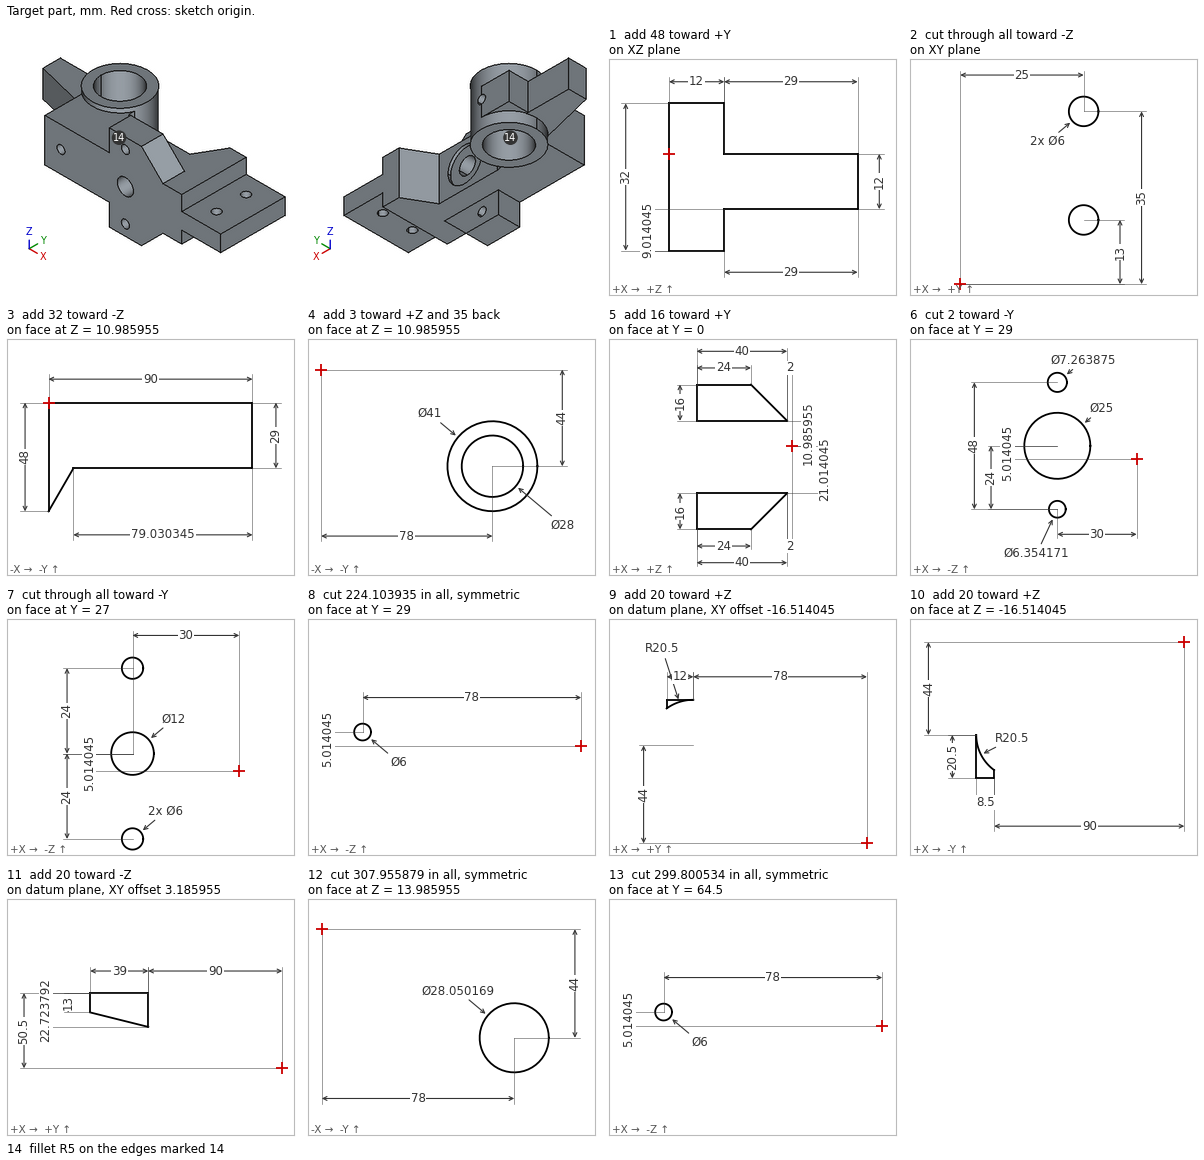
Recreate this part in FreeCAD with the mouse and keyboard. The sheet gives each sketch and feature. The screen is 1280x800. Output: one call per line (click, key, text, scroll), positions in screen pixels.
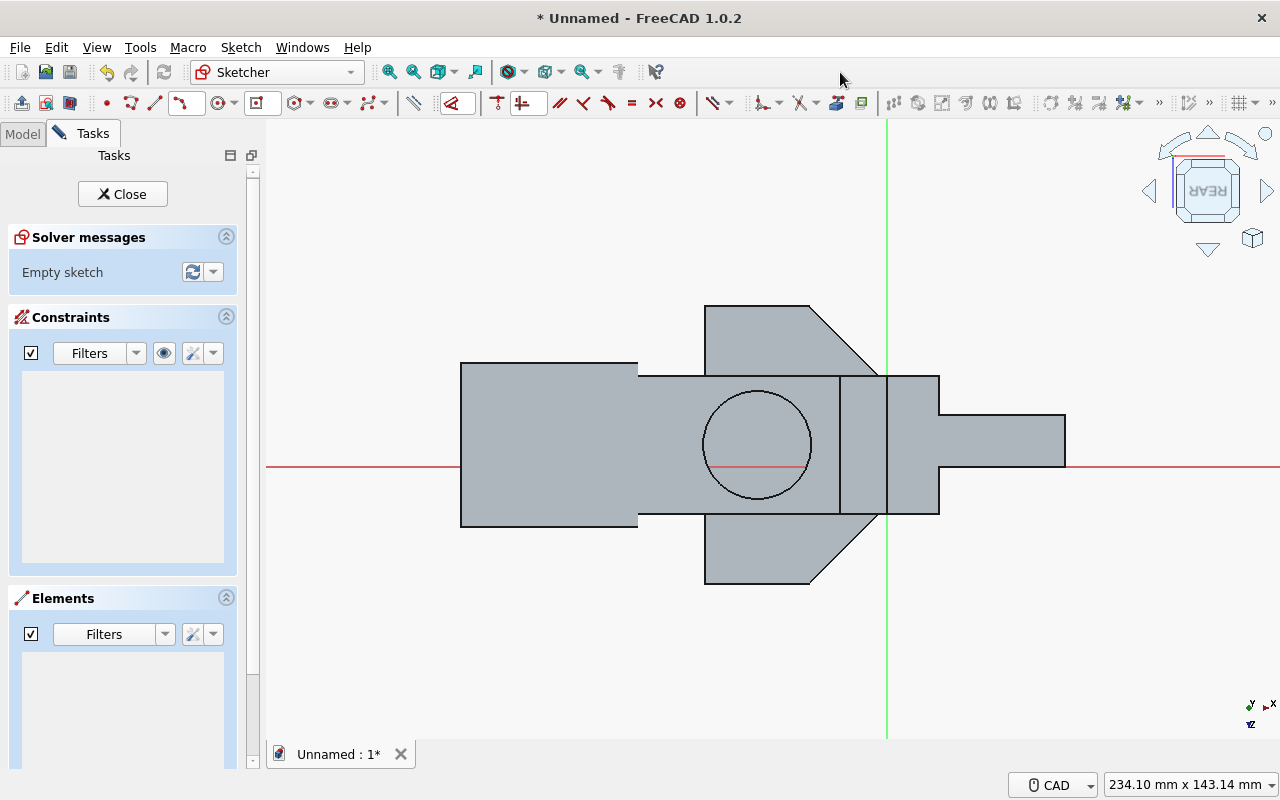
click(70, 104)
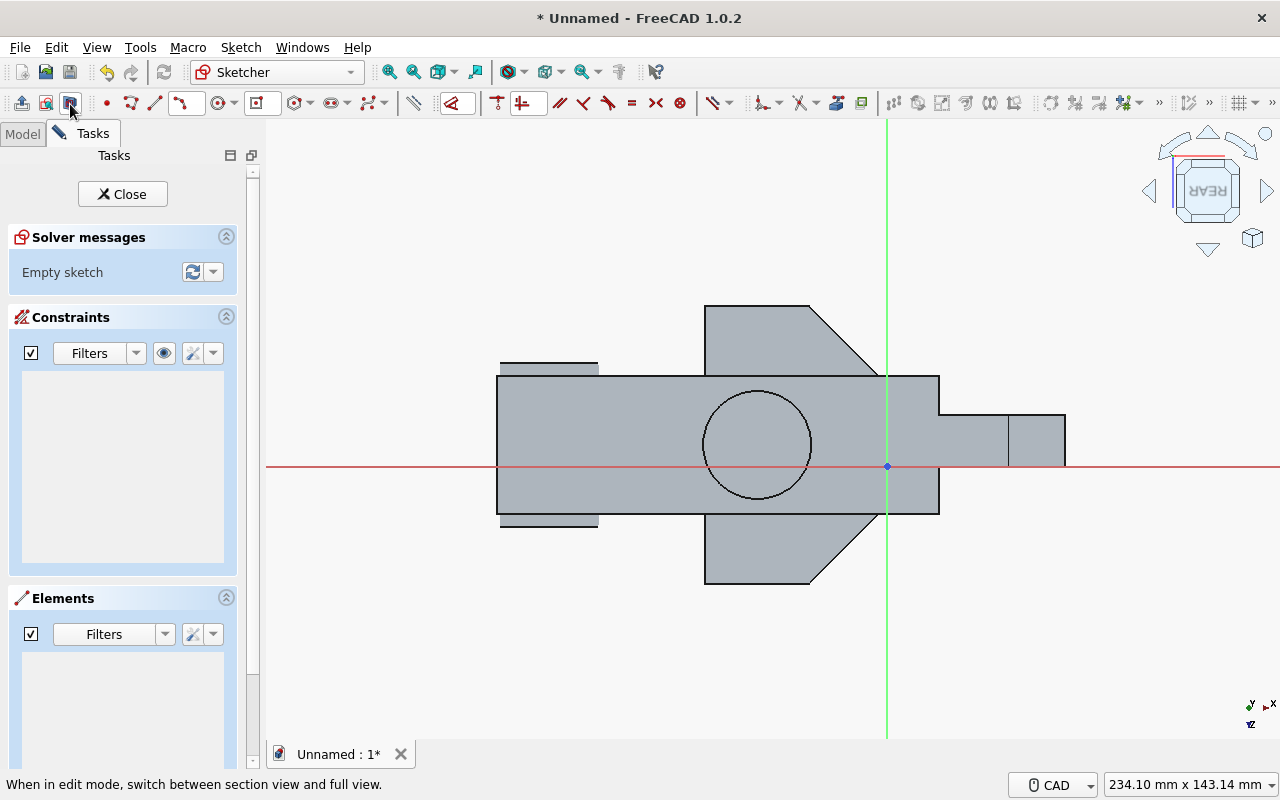
scroll(937, 464, up, 3)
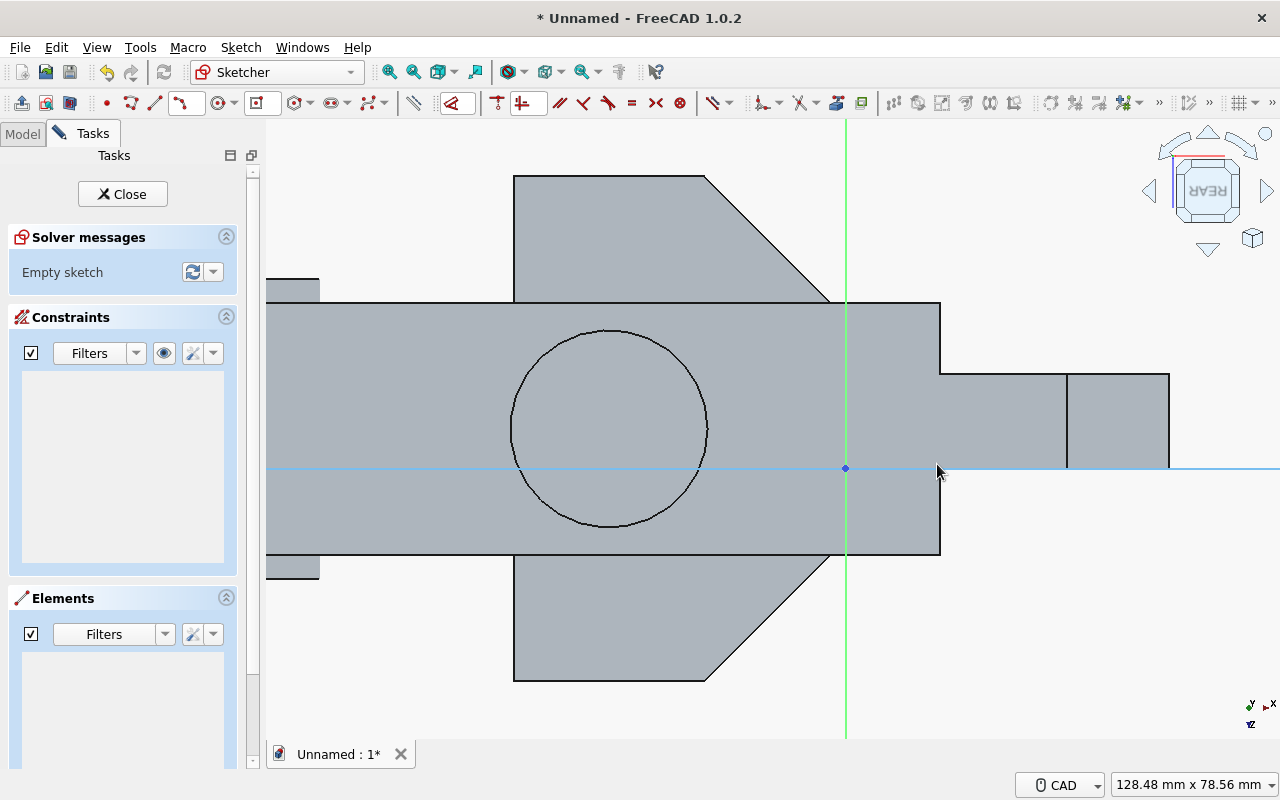
key(g)
key(c)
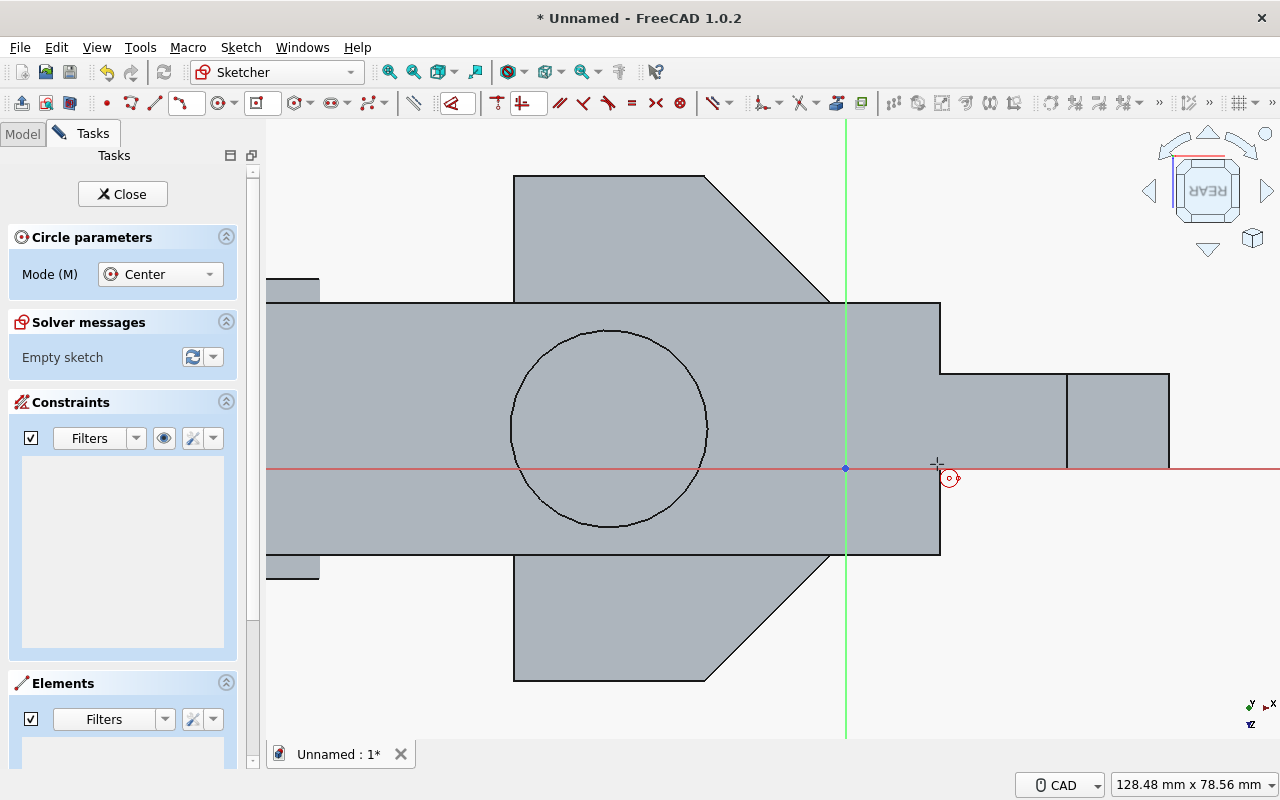
click(609, 429)
move(642, 395)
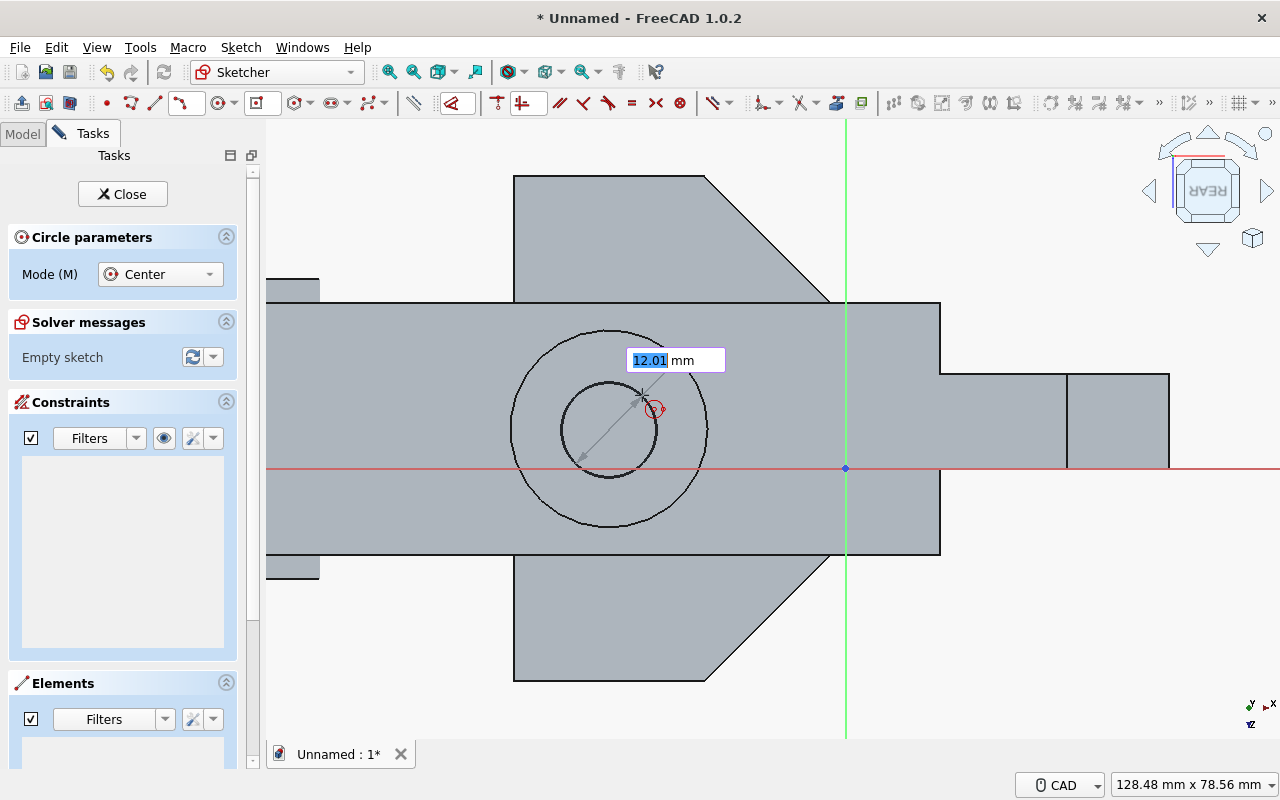
text(12)
key(Return)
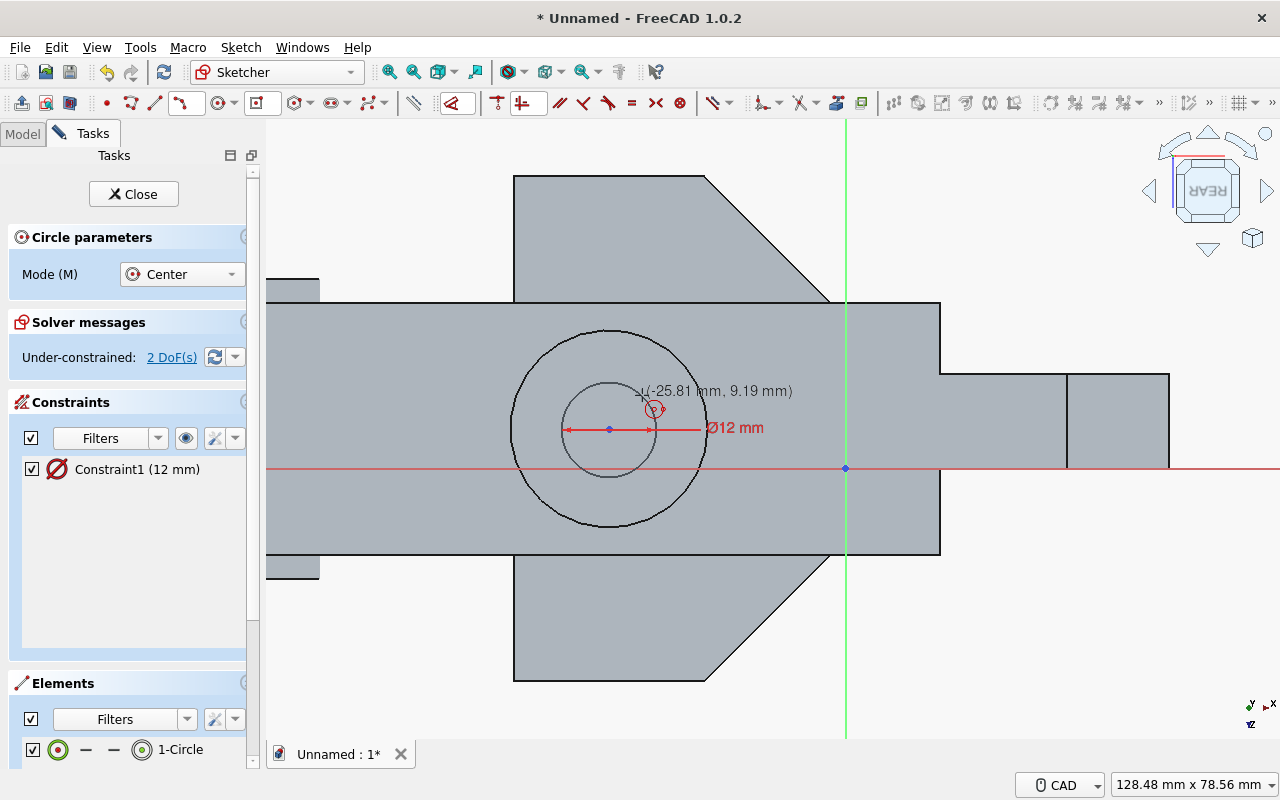
click(609, 618)
move(626, 602)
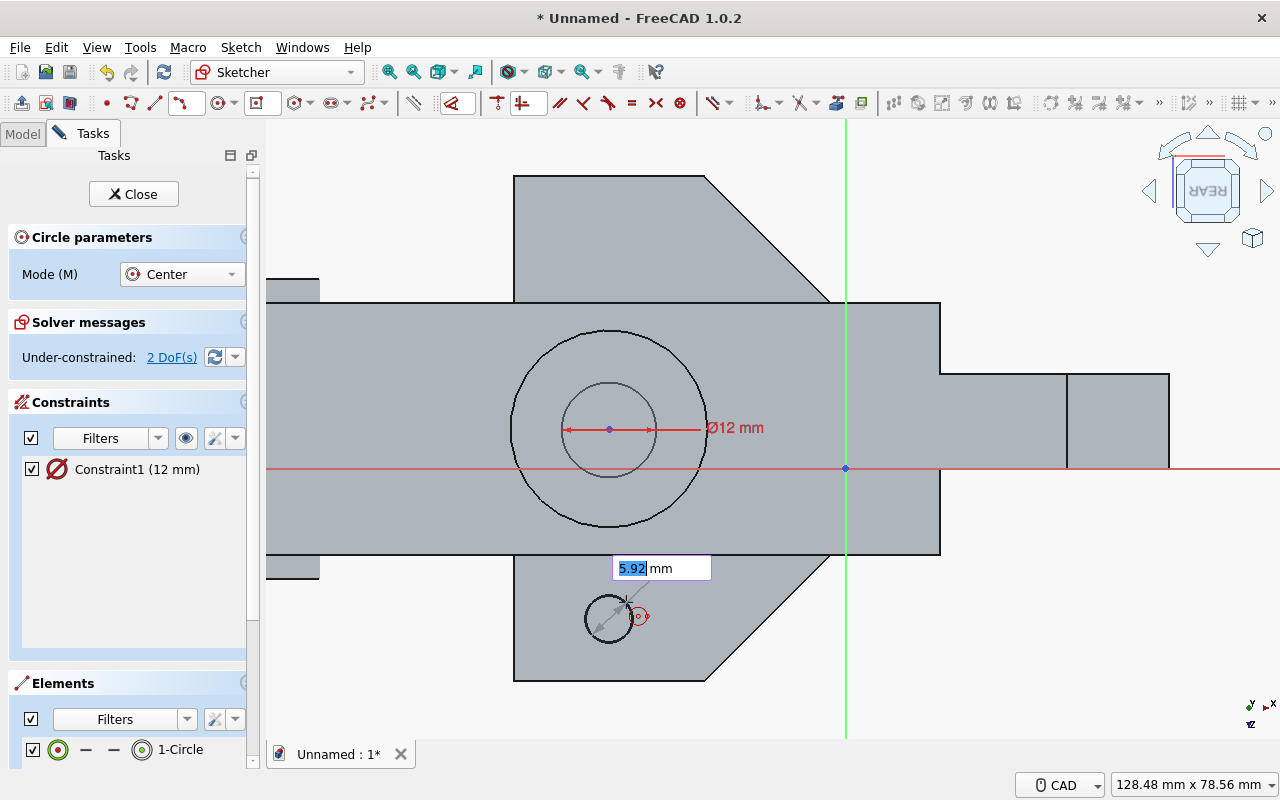
text(6)
key(Return)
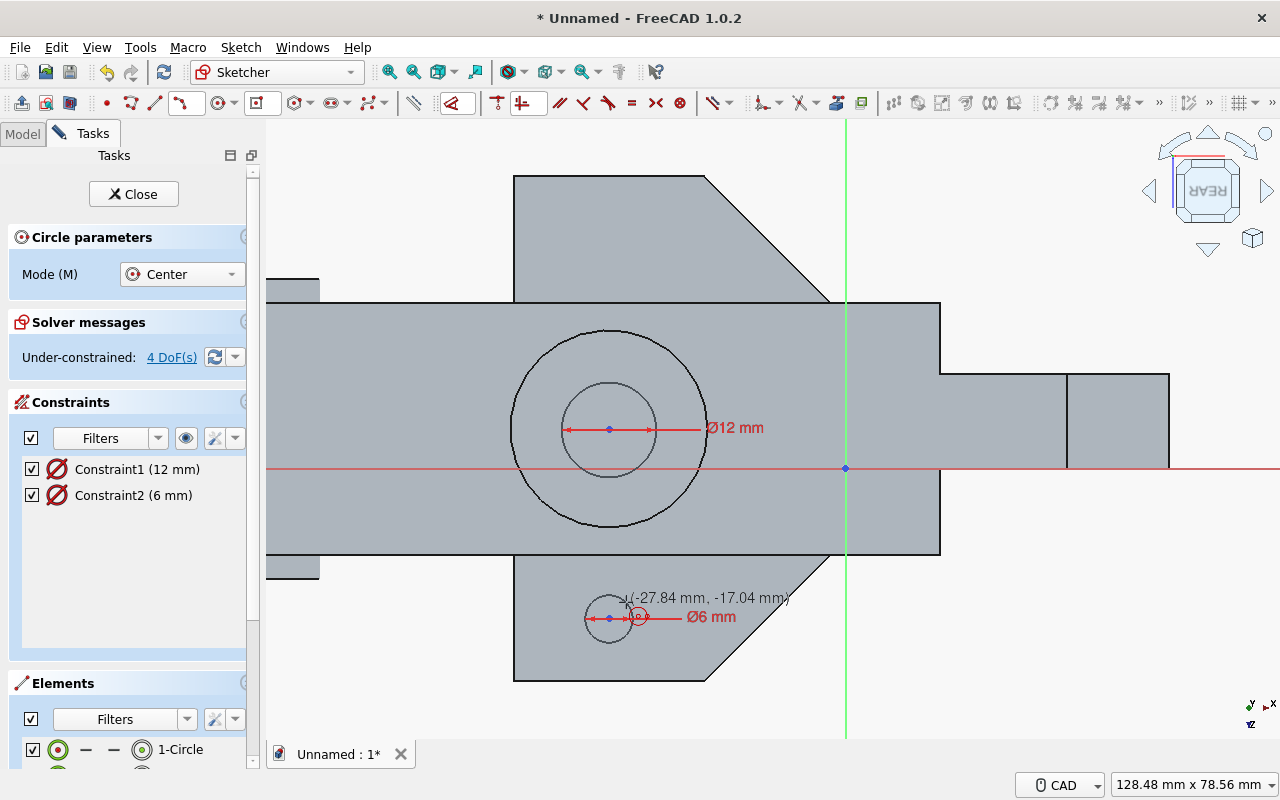
click(609, 240)
move(626, 223)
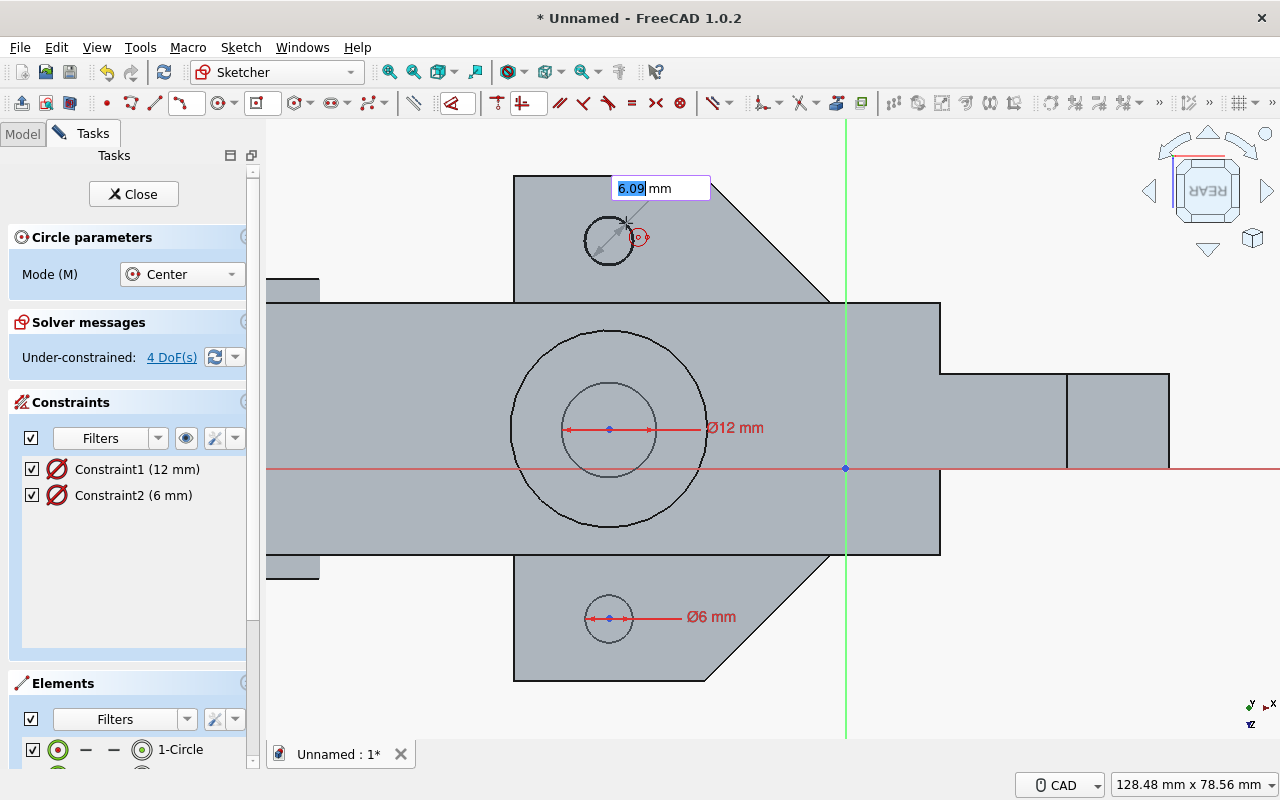
text(6)
key(Return)
key(Escape)